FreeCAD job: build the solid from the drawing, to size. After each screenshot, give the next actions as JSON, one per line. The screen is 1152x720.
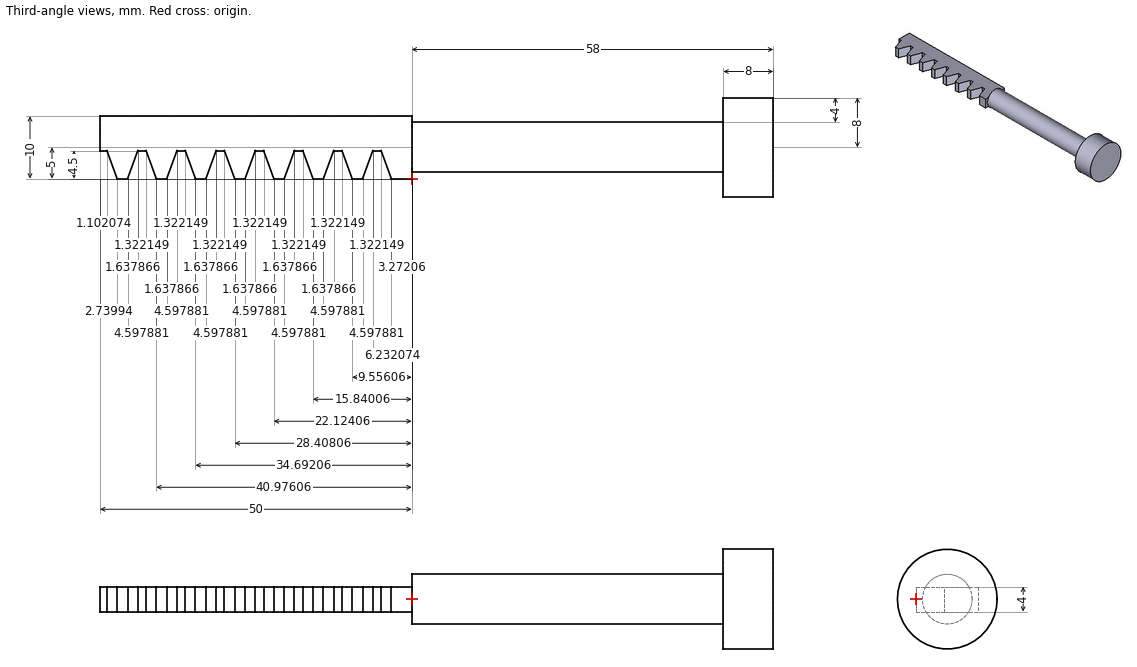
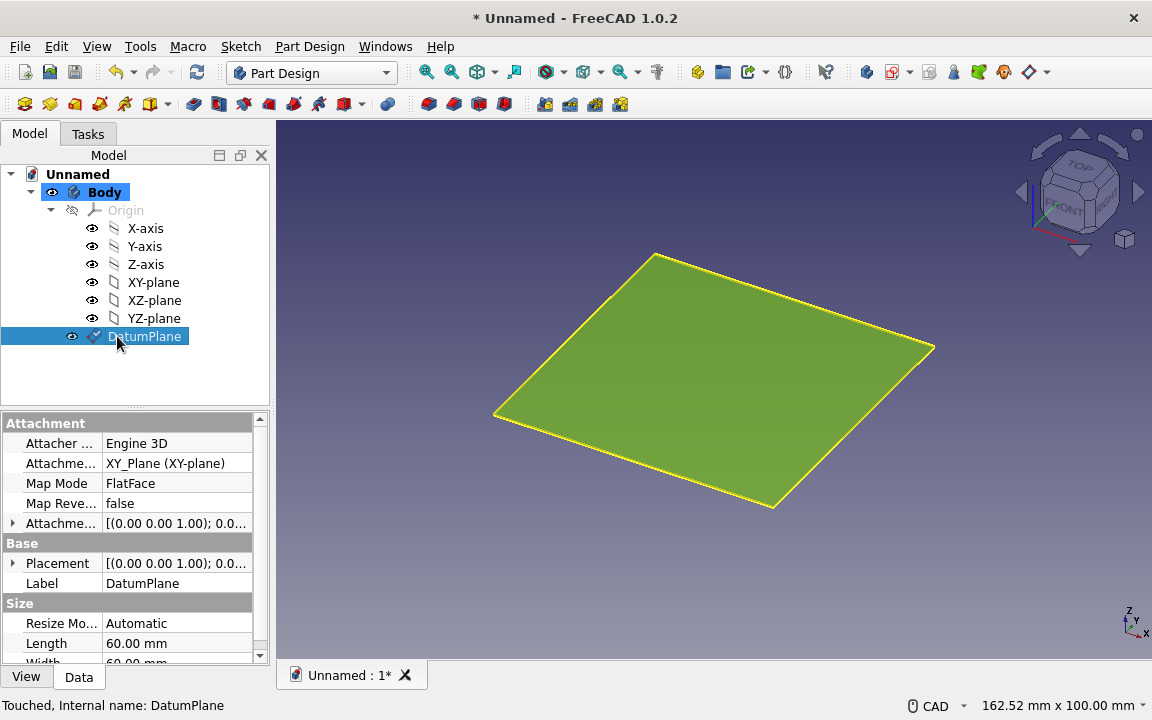
{"action": "left_click", "coordinate": [892, 72]}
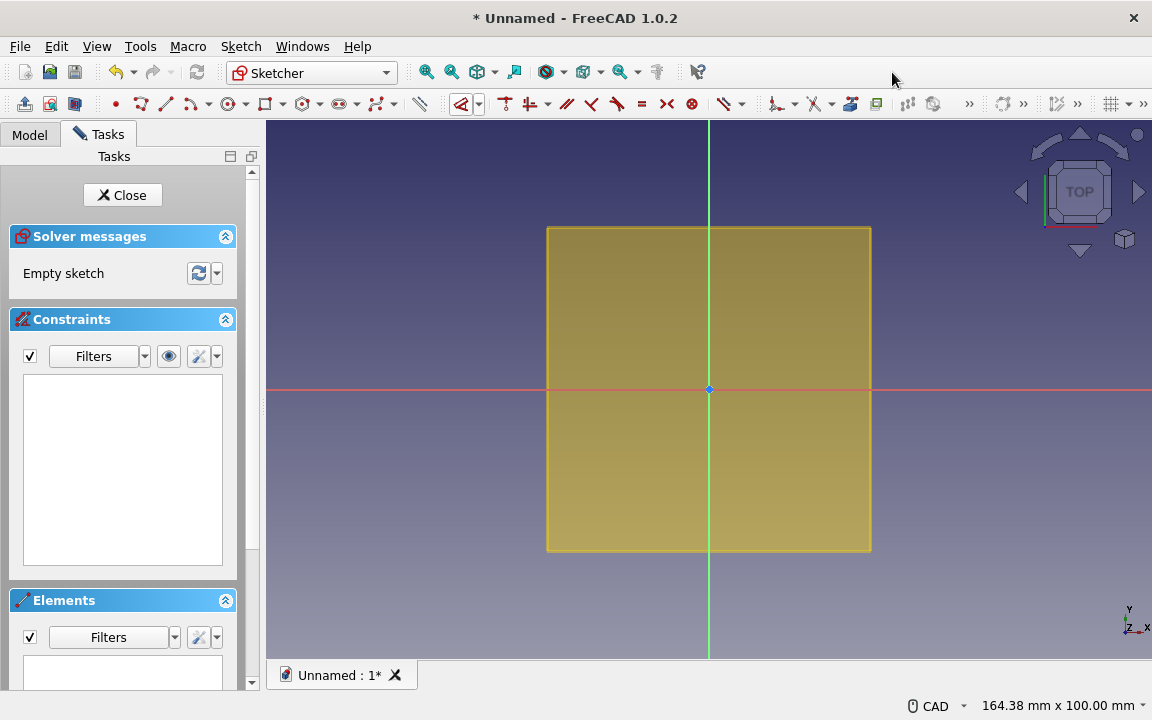
{"action": "scroll", "coordinate": [494, 330], "scroll_direction": "up", "scroll_amount": 3}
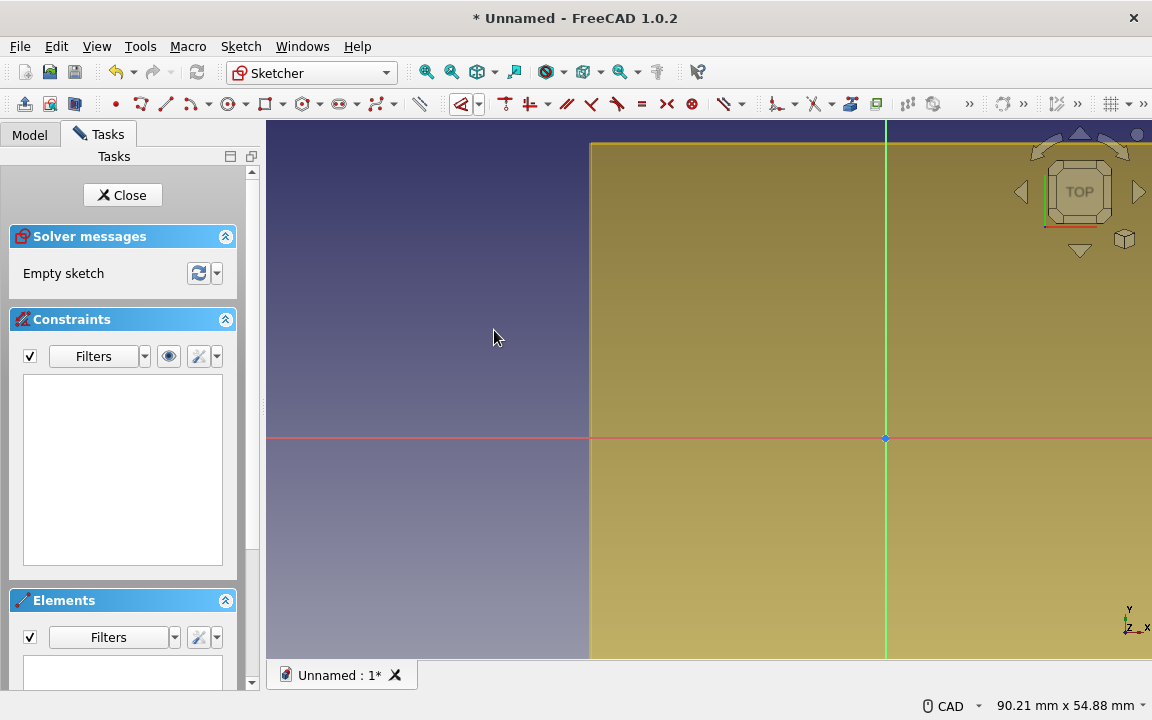
{"action": "left_click", "coordinate": [264, 104]}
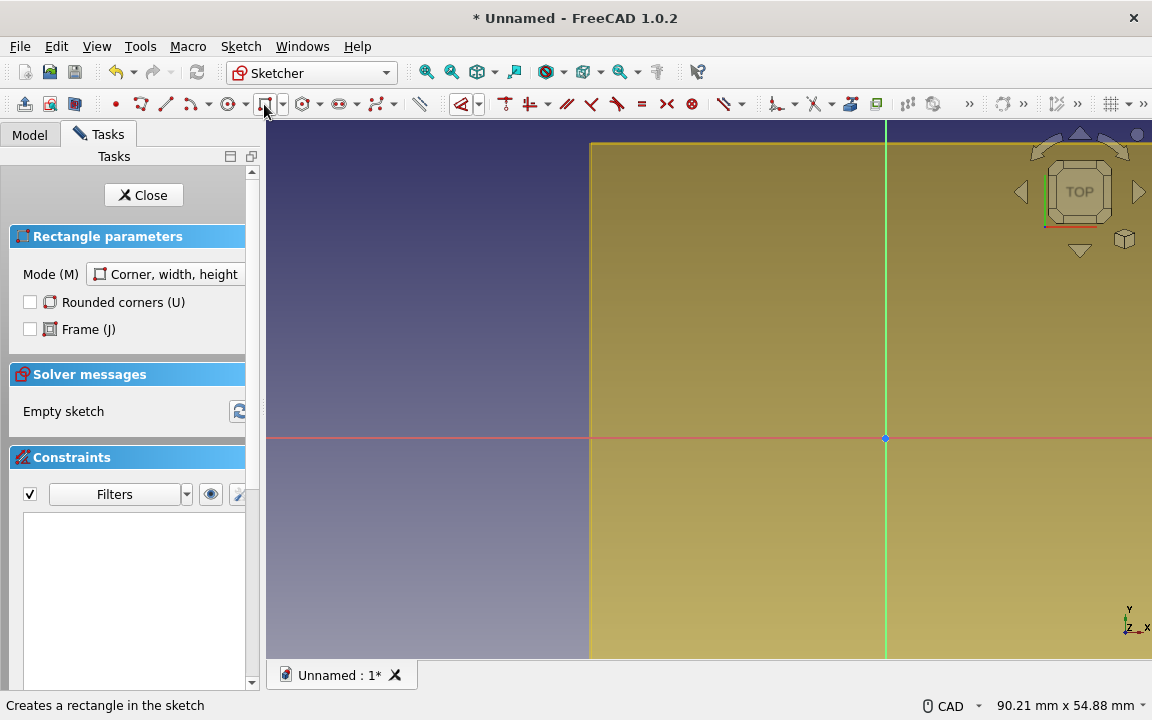
{"action": "left_click", "coordinate": [886, 438]}
{"action": "mouse_move", "coordinate": [394, 340]}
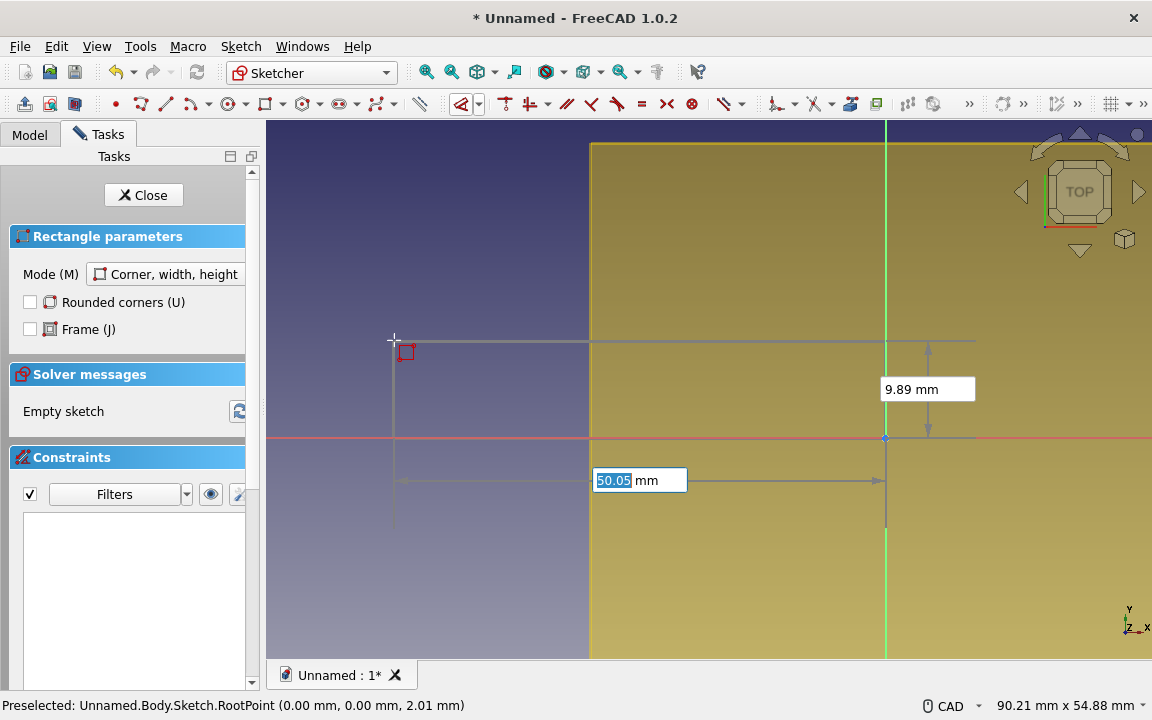
{"action": "type", "text": "50"}
{"action": "key", "text": "Tab"}
{"action": "type", "text": "10"}
{"action": "key", "text": "Return"}
{"action": "key", "text": "Escape"}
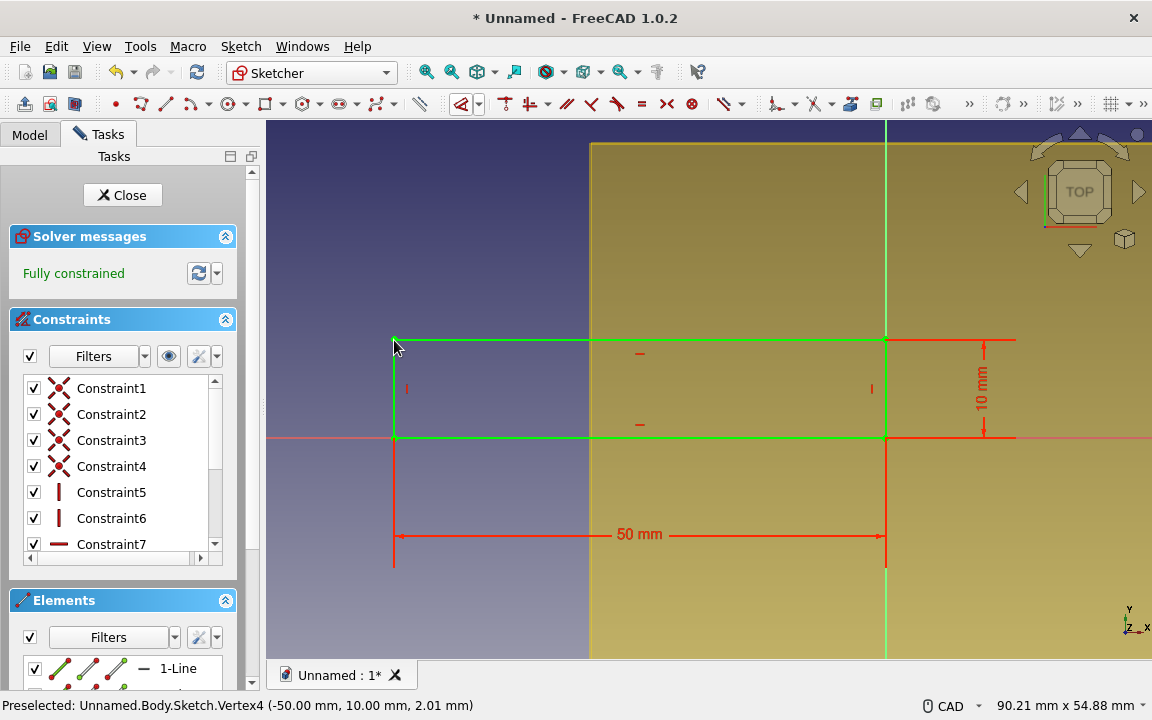
{"action": "left_click", "coordinate": [123, 195]}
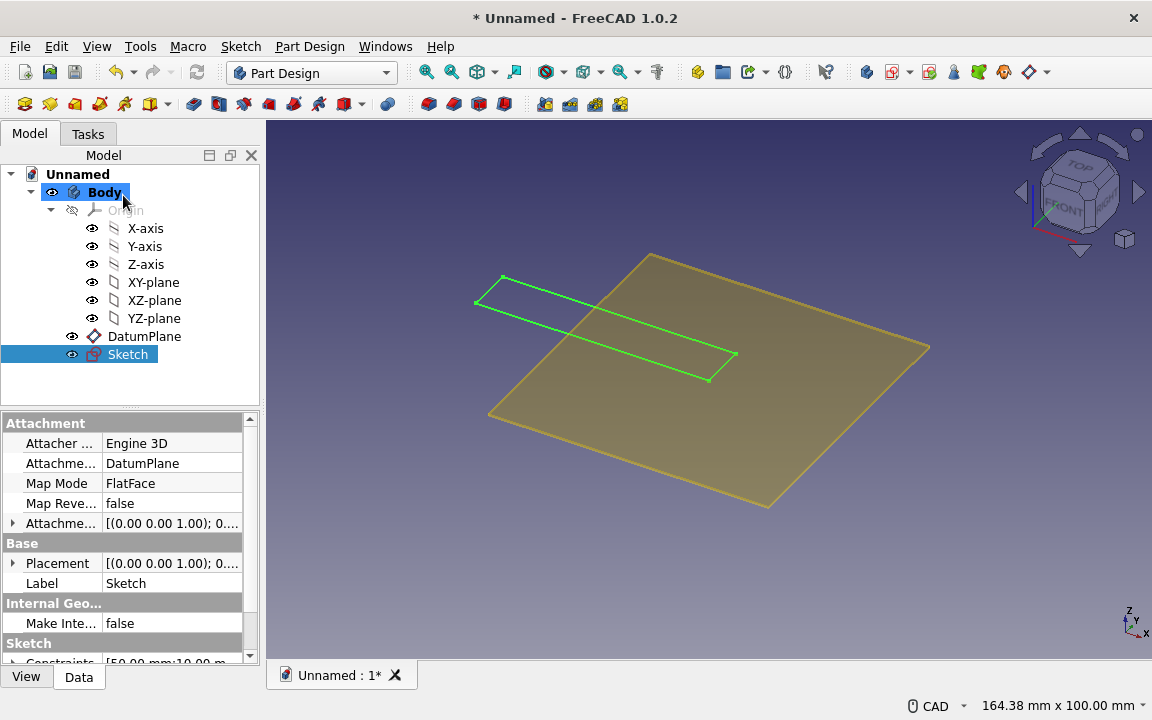
{"action": "left_click", "coordinate": [25, 104]}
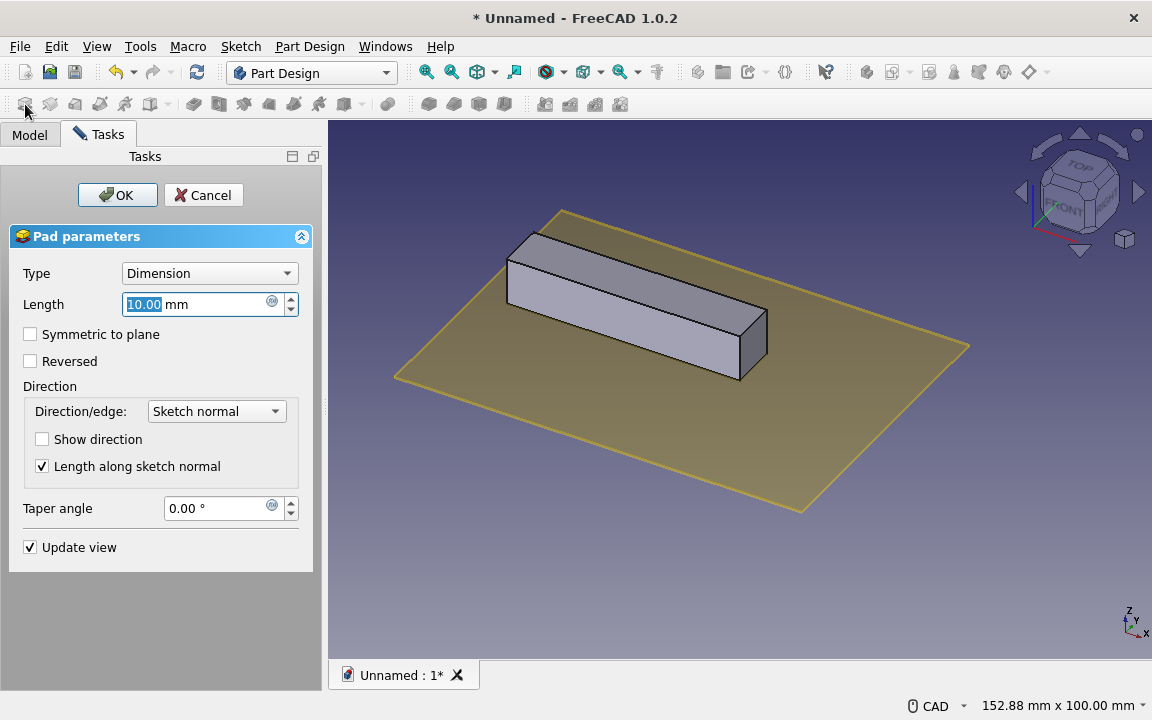
{"action": "type", "text": "4"}
{"action": "key", "text": "Tab"}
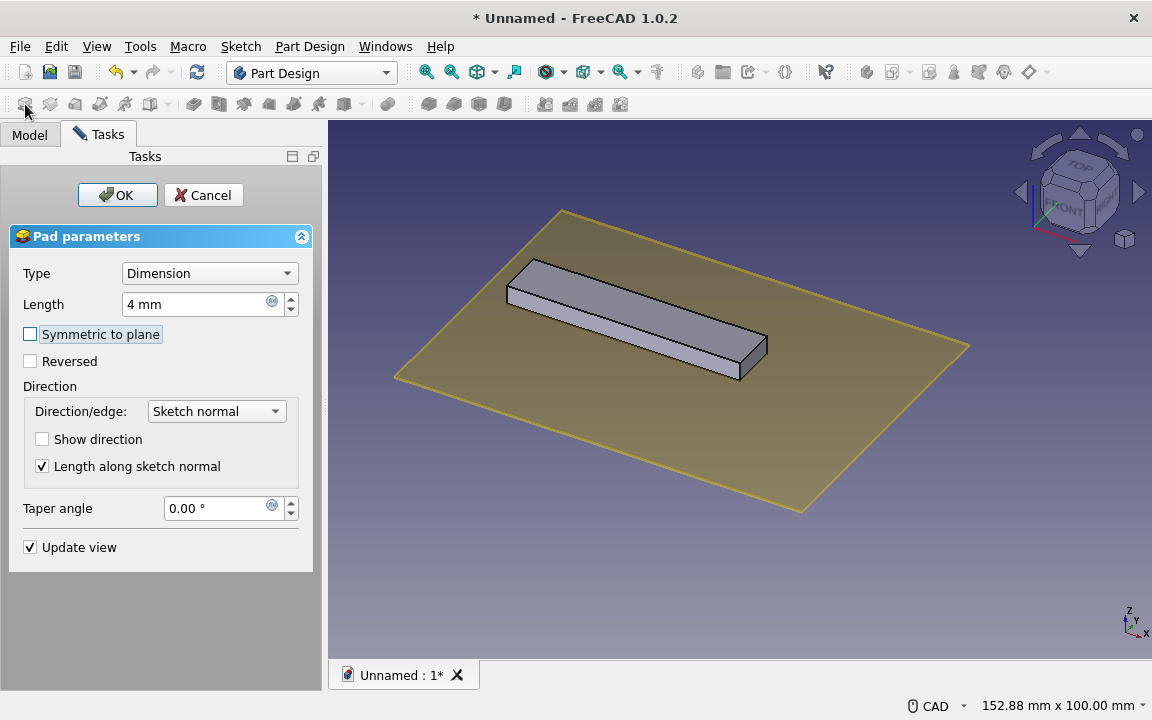
{"action": "left_click", "coordinate": [31, 361]}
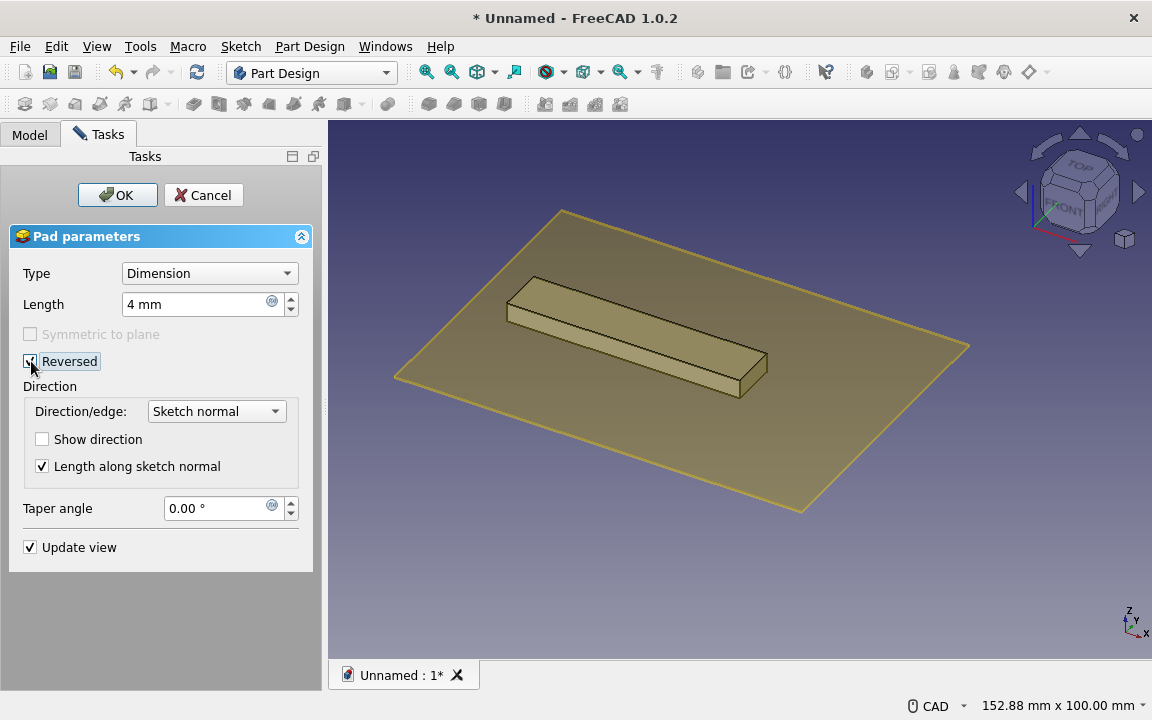
{"action": "left_click", "coordinate": [118, 195]}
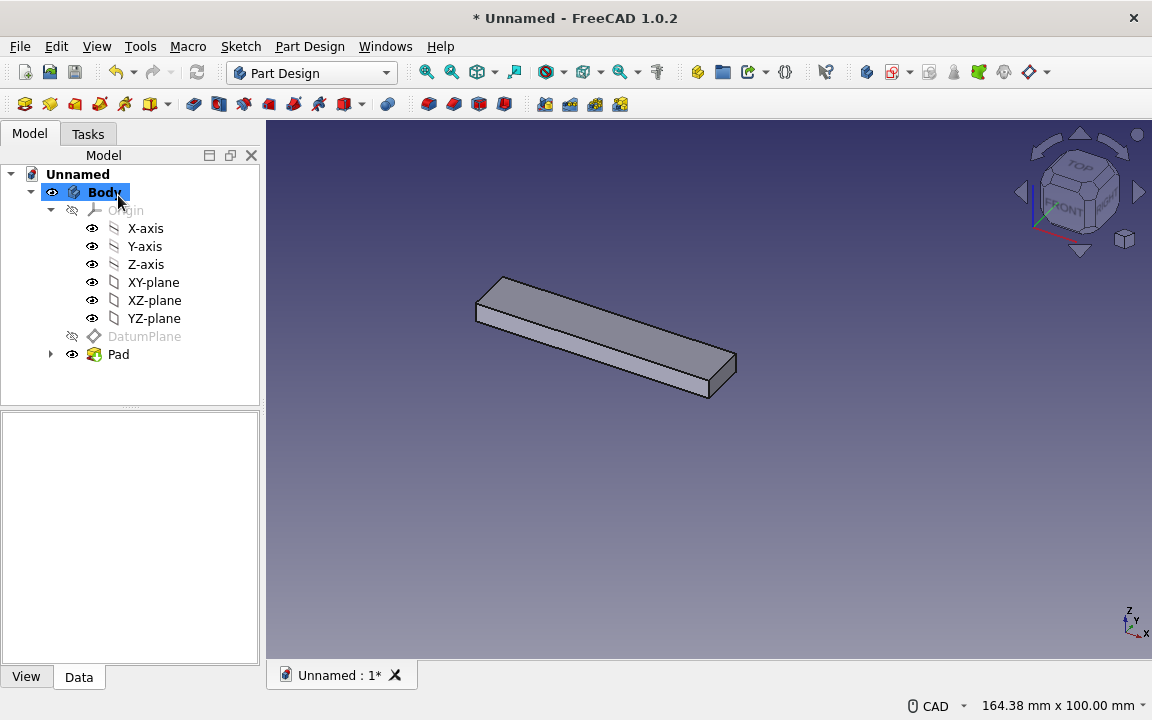
{"action": "left_click", "coordinate": [427, 72]}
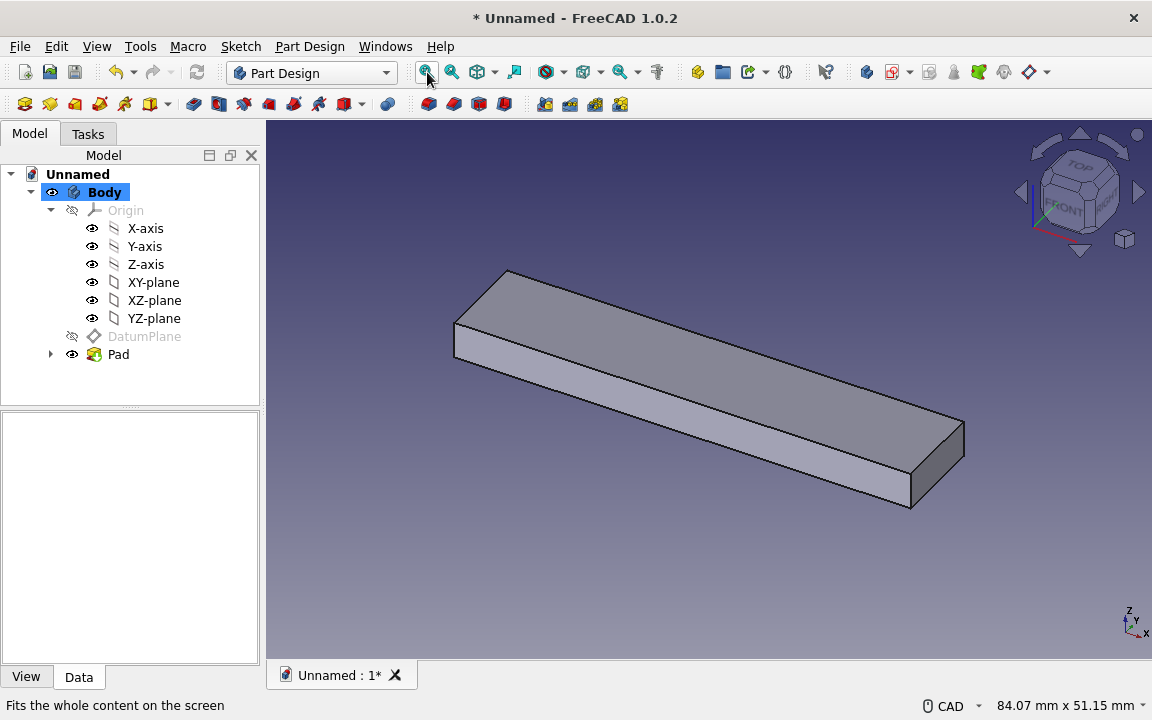
{"action": "key", "text": "5"}